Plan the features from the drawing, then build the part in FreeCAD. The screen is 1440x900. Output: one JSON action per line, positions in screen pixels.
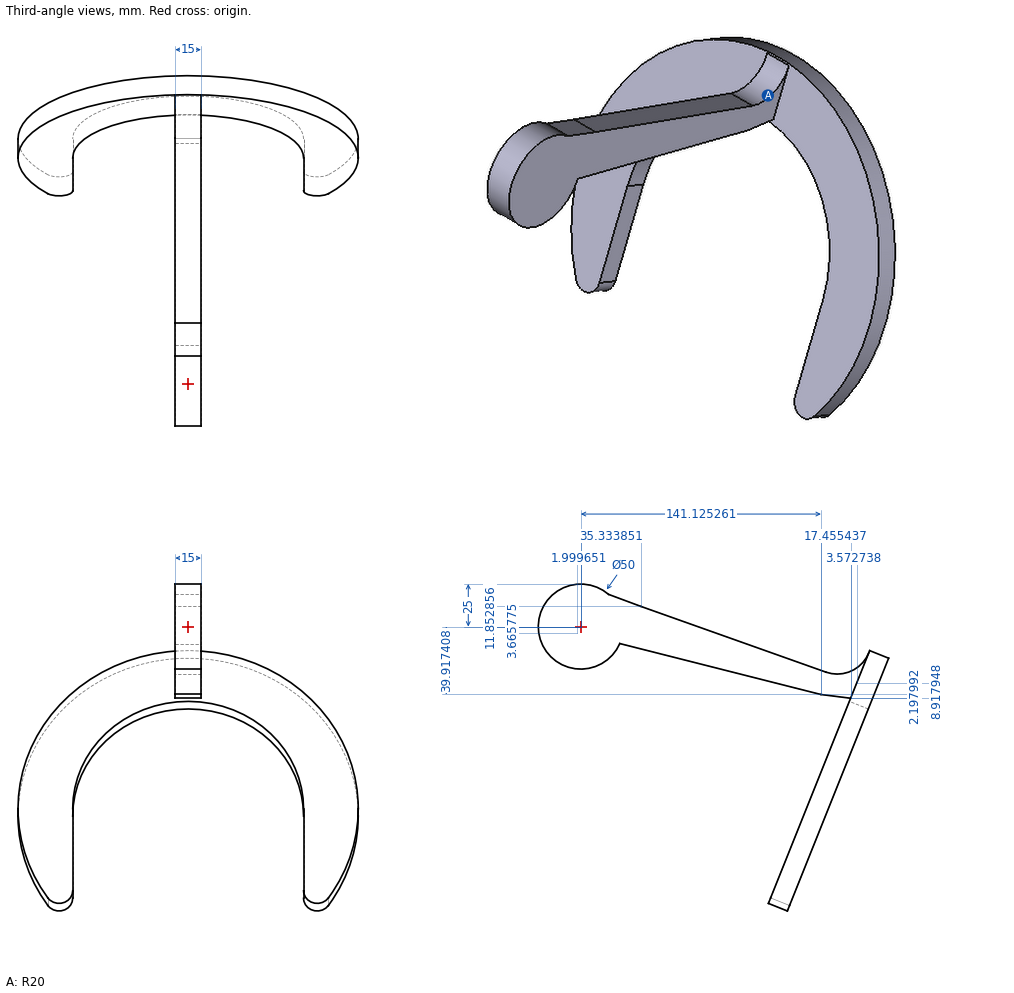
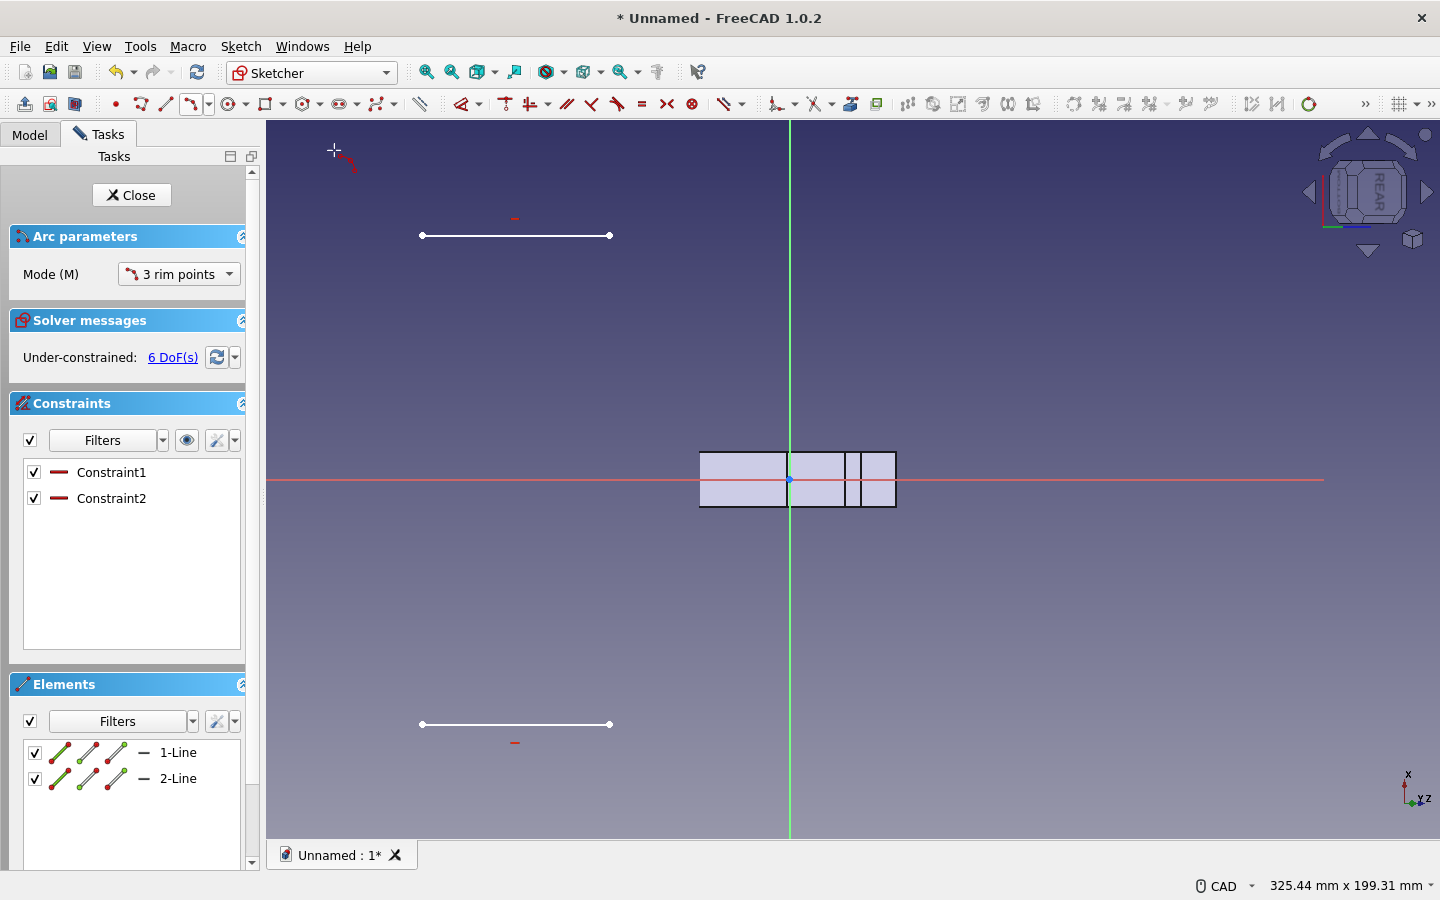
{"action": "left_click", "coordinate": [609, 236]}
{"action": "left_click", "coordinate": [609, 725]}
{"action": "left_click", "coordinate": [842, 555]}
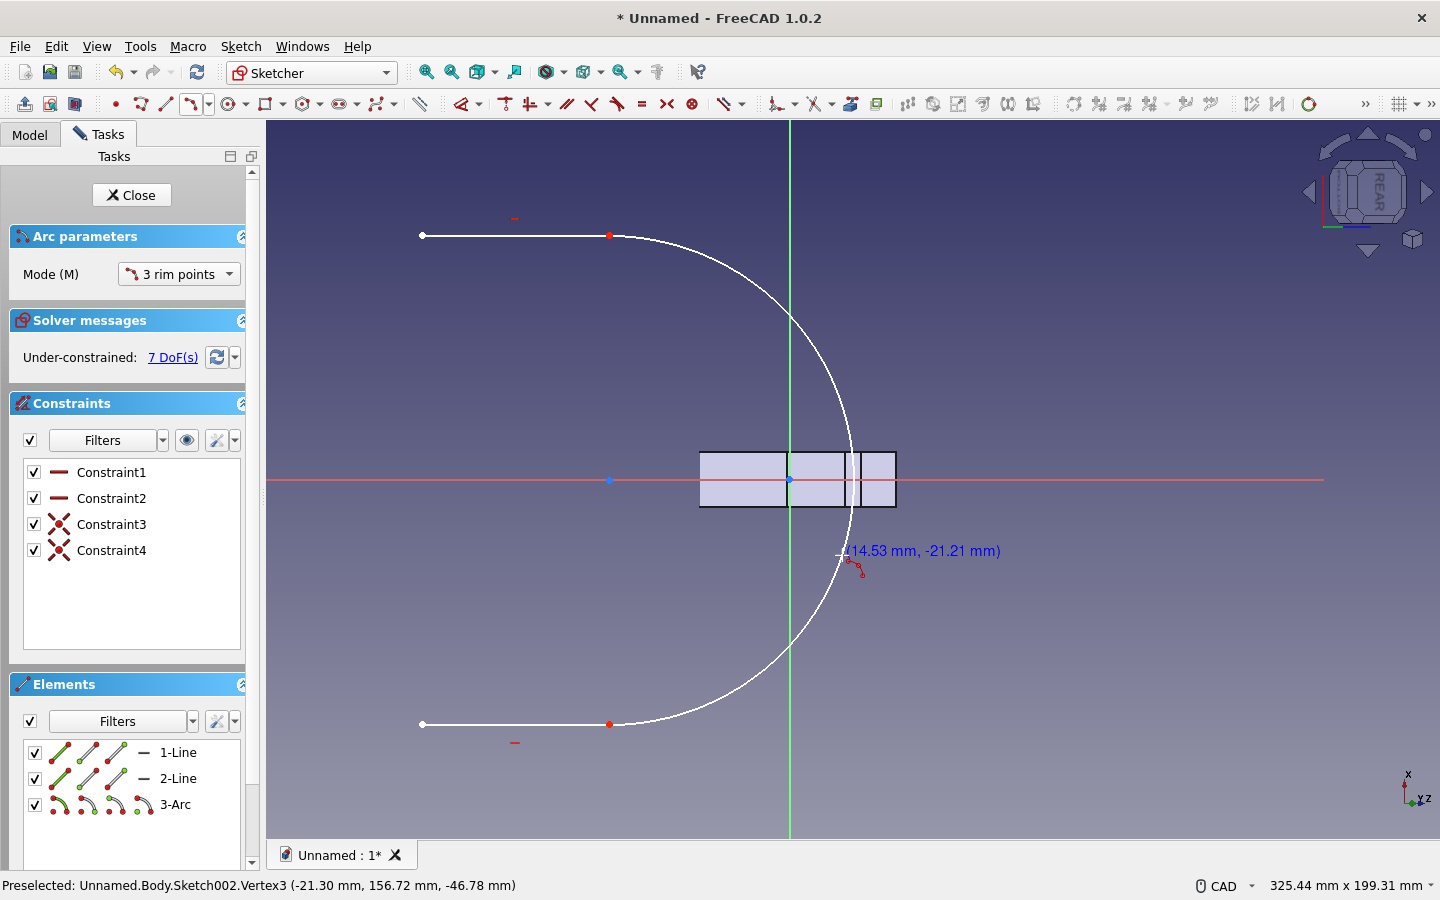
{"action": "left_click", "coordinate": [422, 725]}
{"action": "left_click", "coordinate": [405, 777]}
{"action": "left_click", "coordinate": [394, 745]}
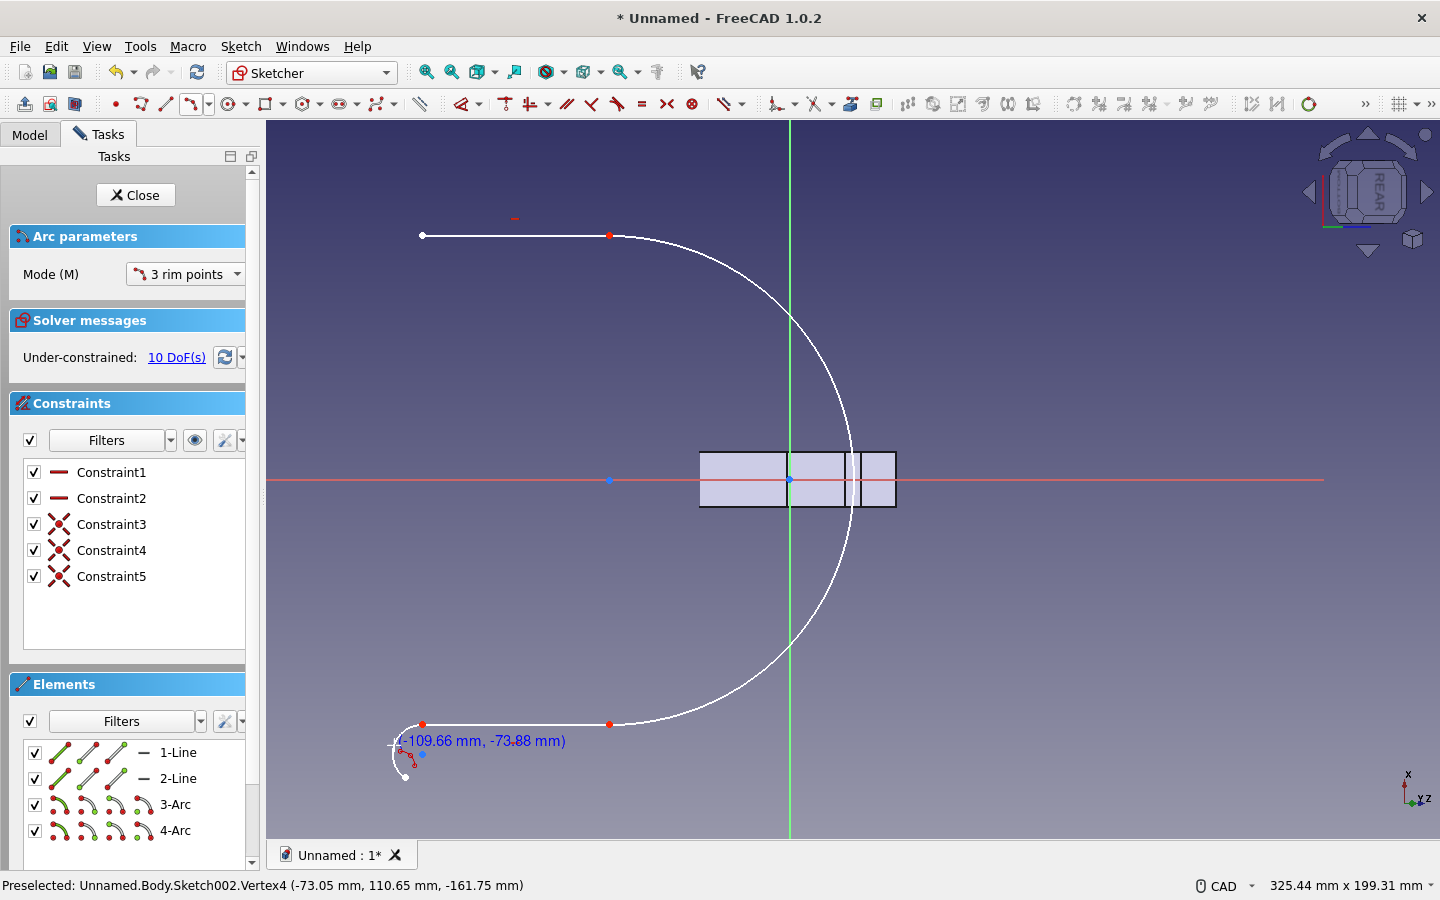
{"action": "left_click", "coordinate": [405, 778]}
{"action": "left_click", "coordinate": [405, 182]}
{"action": "left_click", "coordinate": [937, 631]}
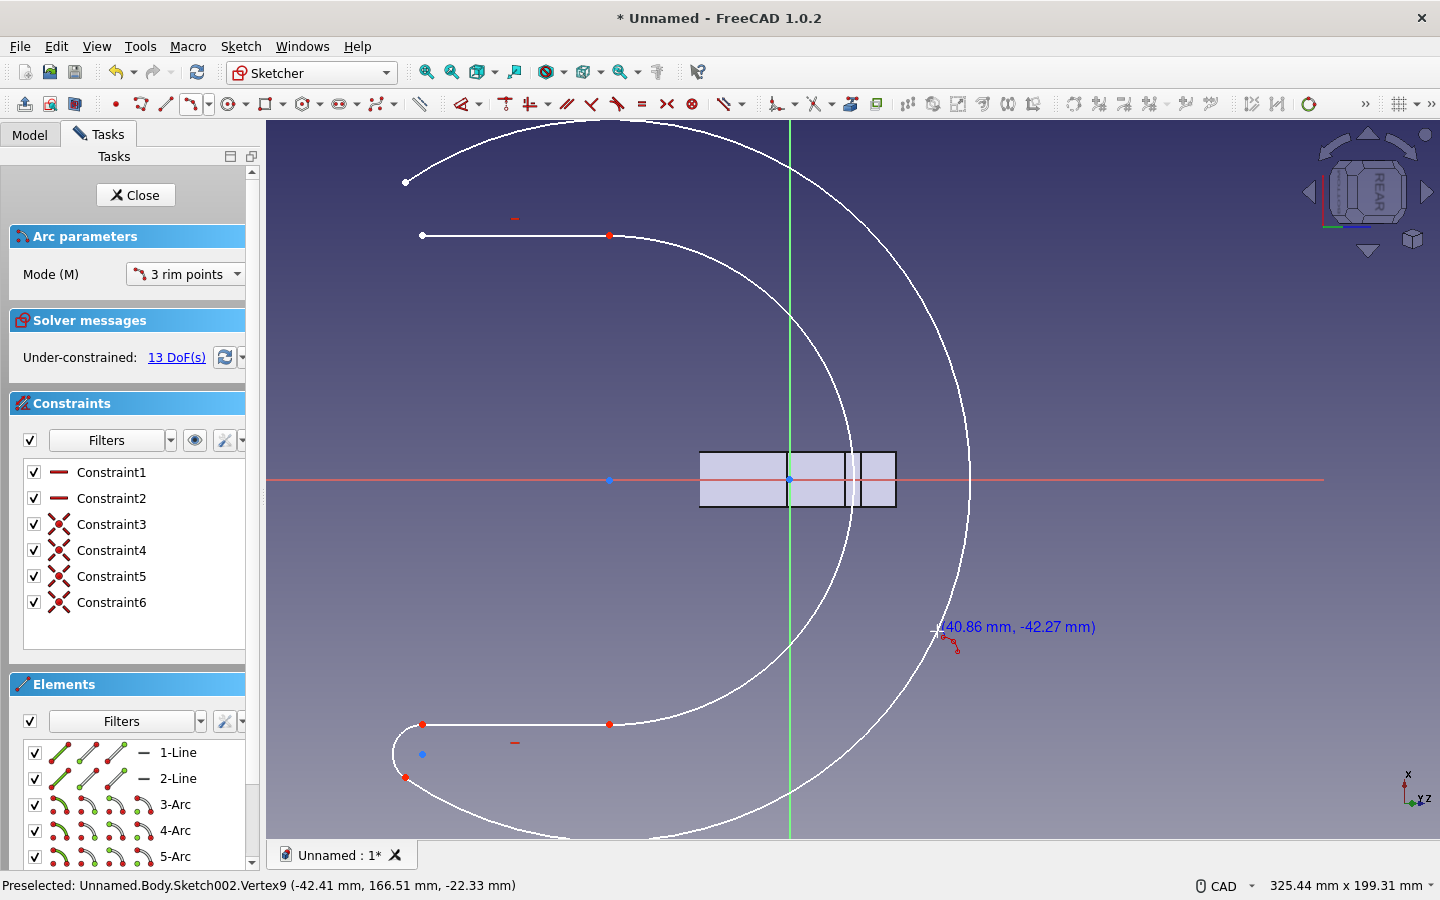
{"action": "left_click", "coordinate": [405, 183]}
{"action": "left_click", "coordinate": [422, 236]}
{"action": "left_click", "coordinate": [394, 214]}
{"action": "key", "text": "Escape"}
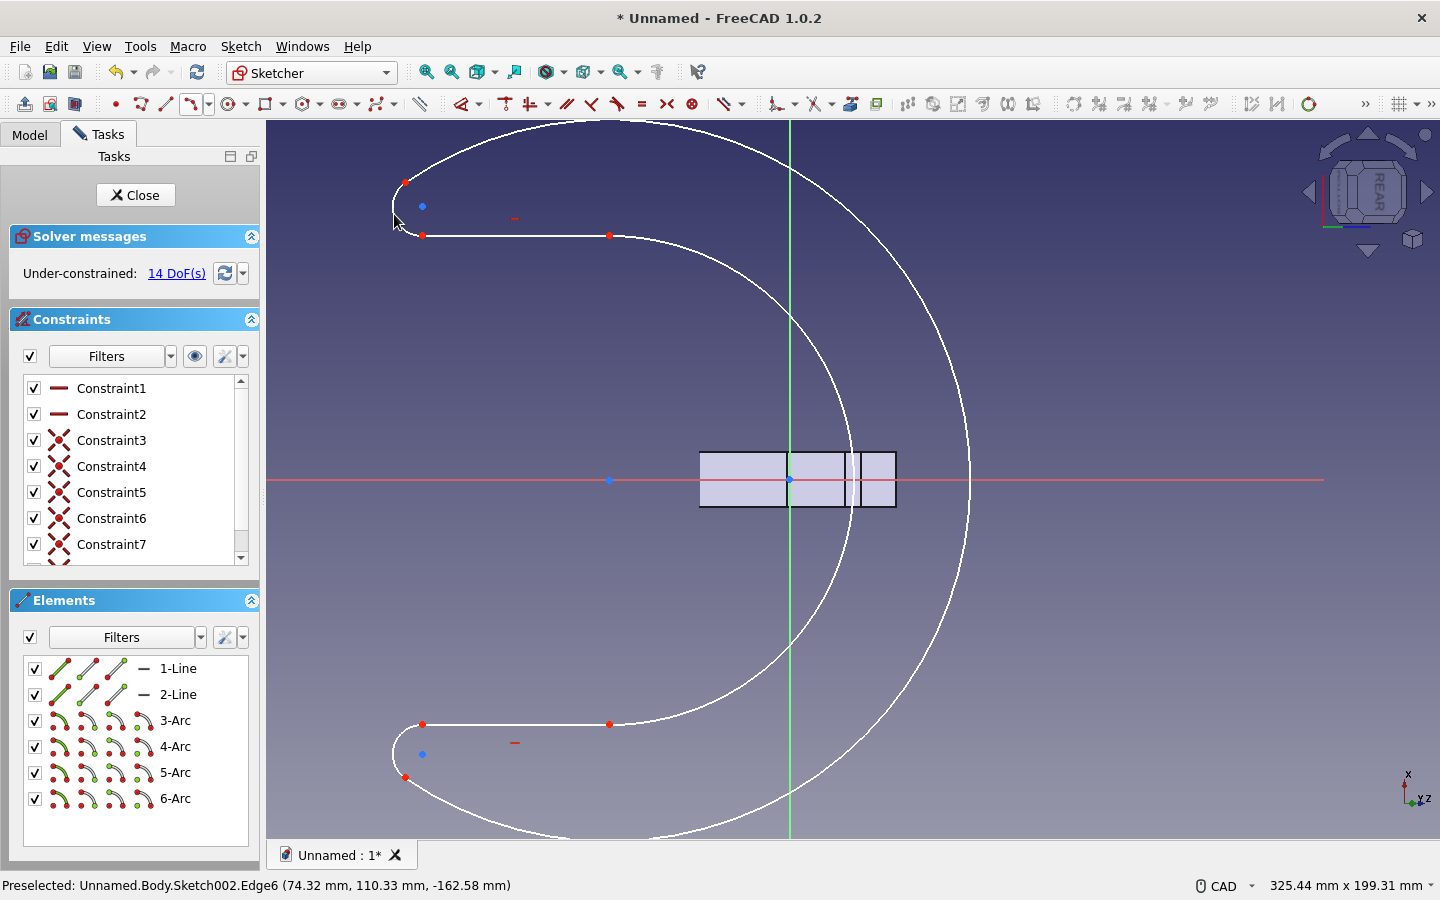
{"action": "left_click", "coordinate": [478, 236]}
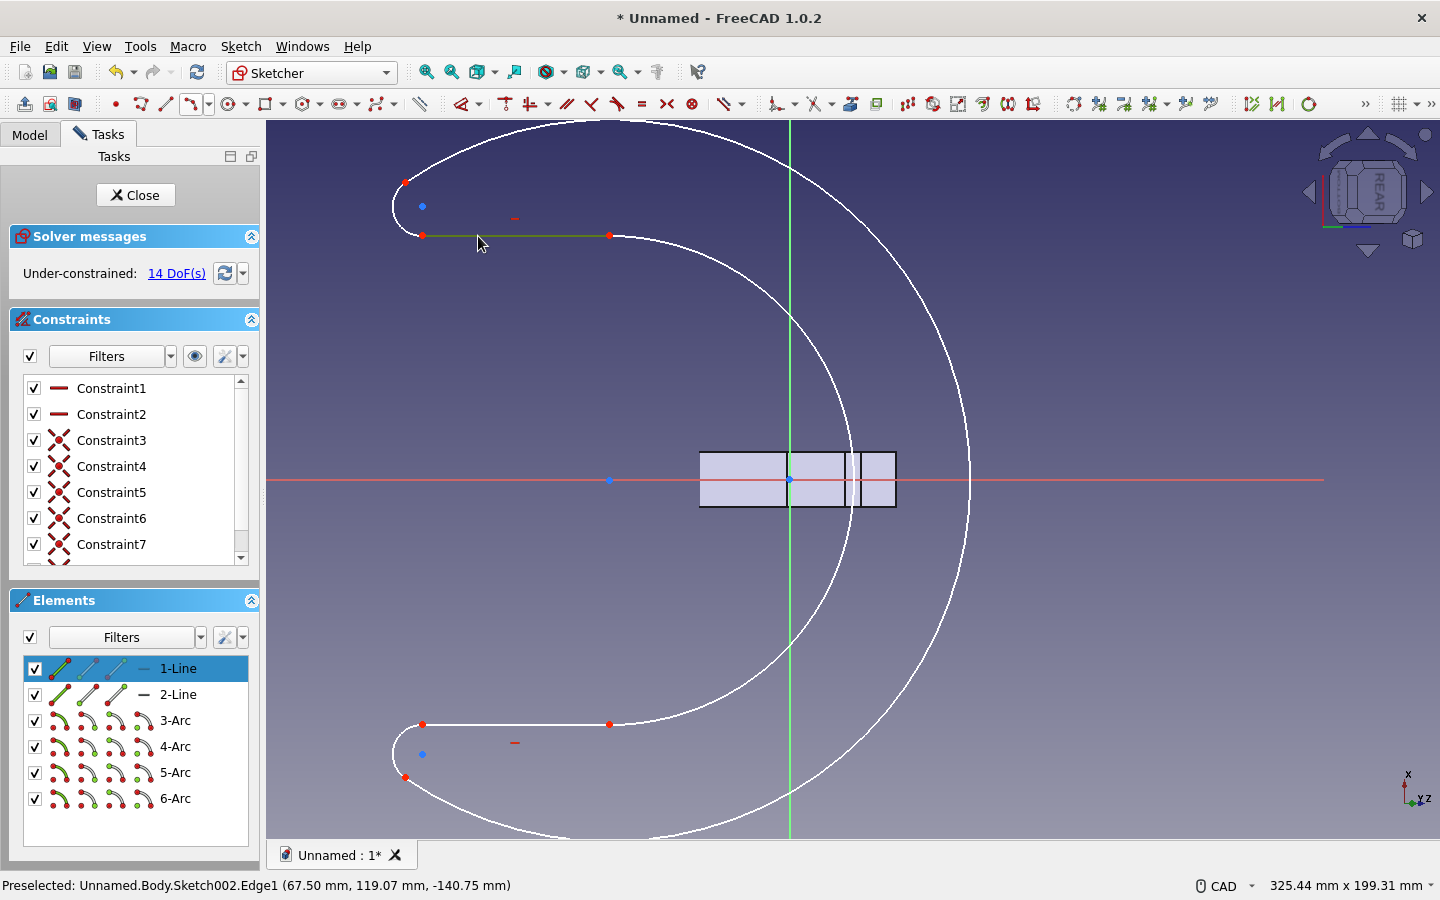
{"action": "left_click", "coordinate": [393, 201]}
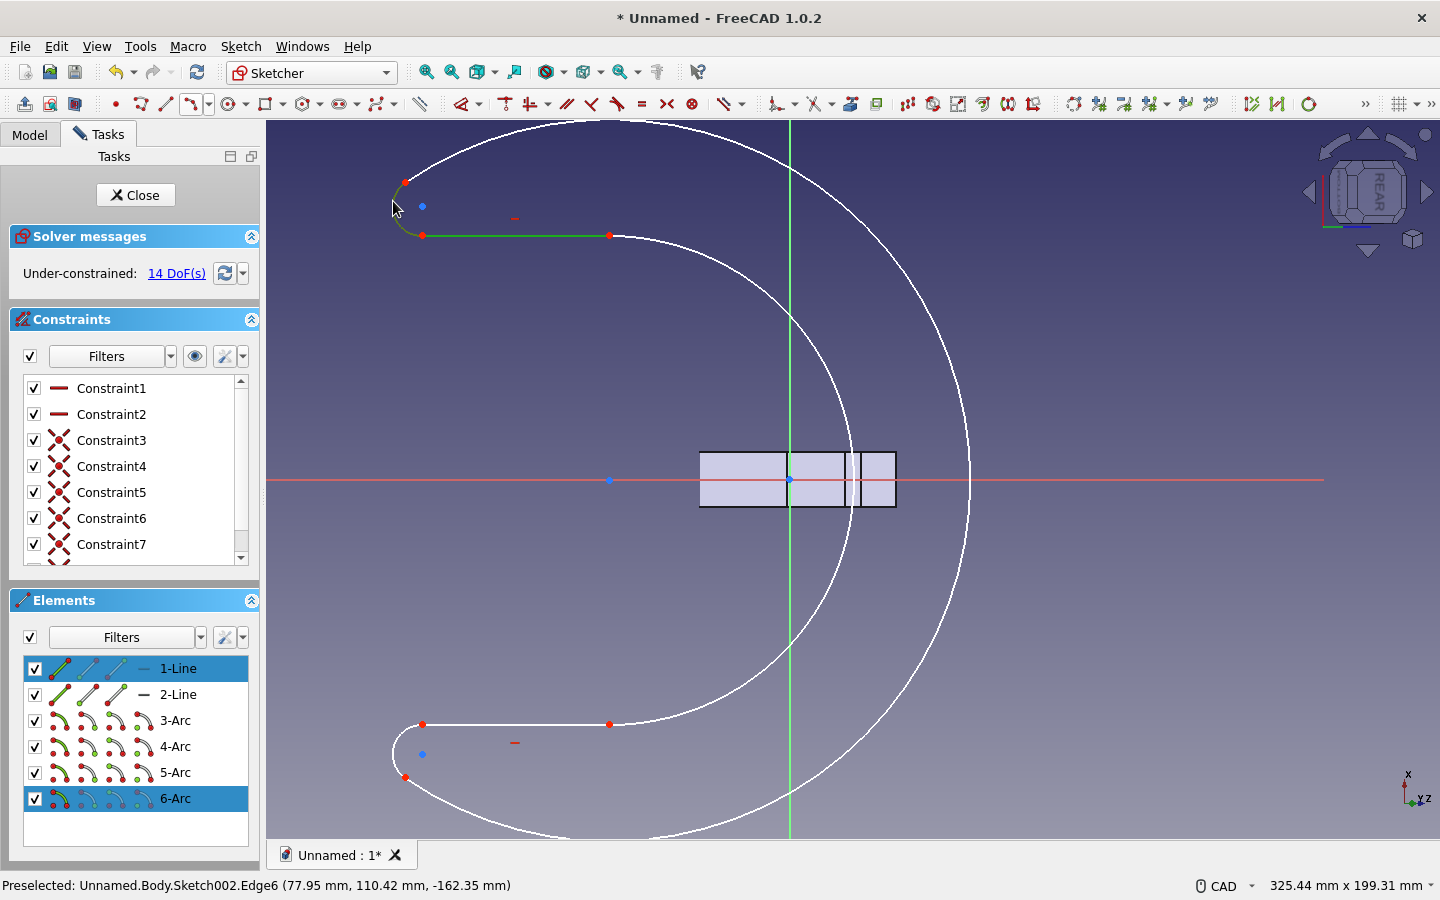
{"action": "key", "text": "t"}